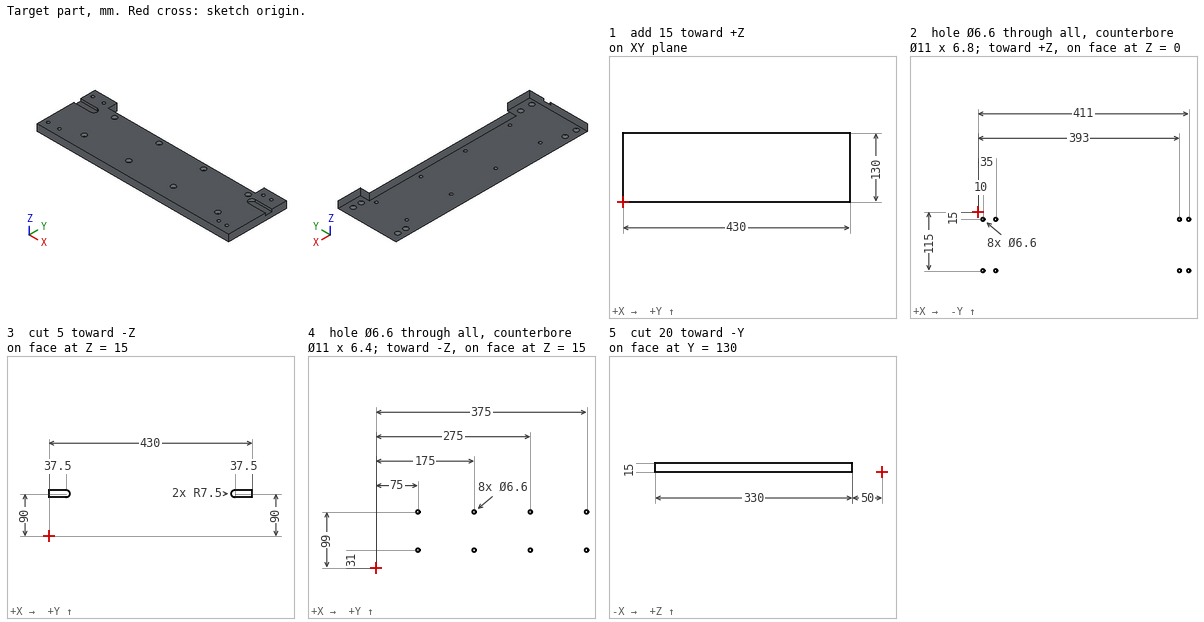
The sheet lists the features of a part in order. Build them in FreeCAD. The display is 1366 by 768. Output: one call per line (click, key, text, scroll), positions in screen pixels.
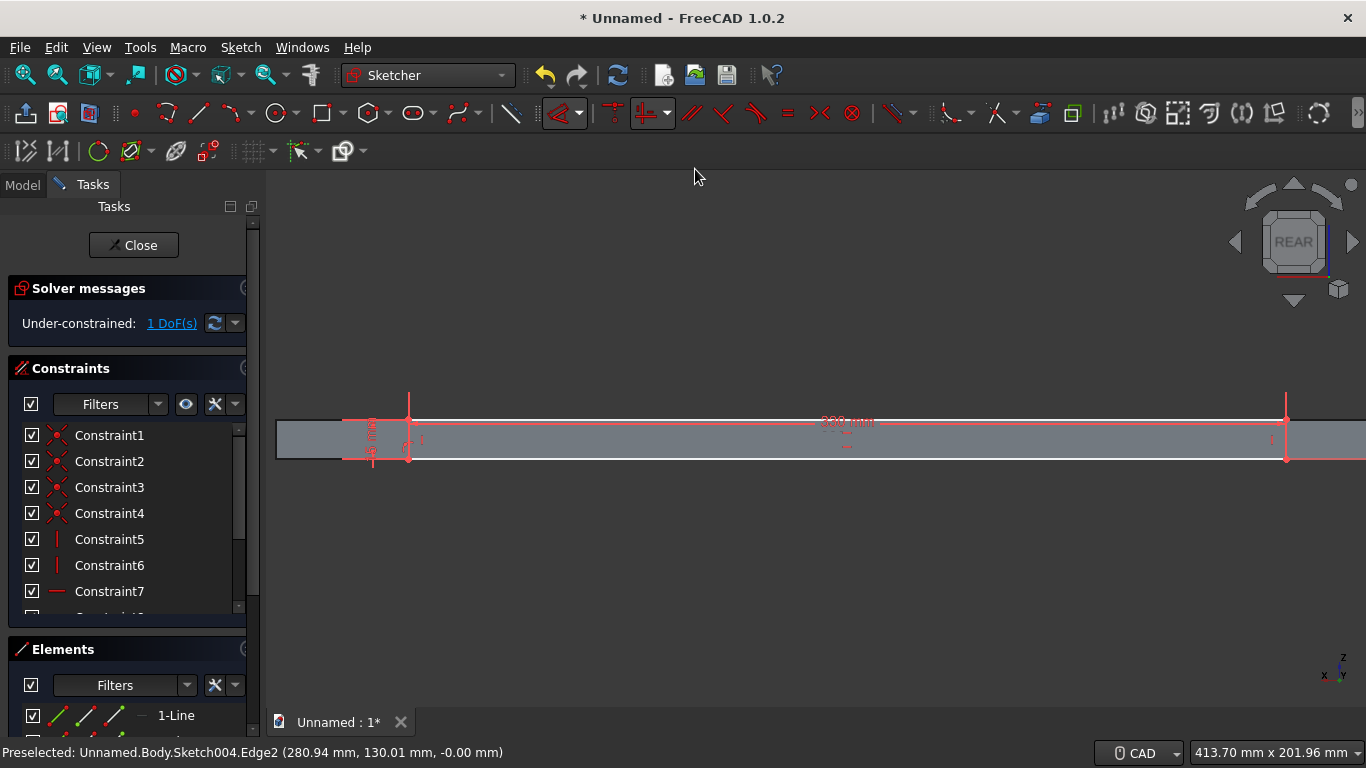
scroll(409, 436, down, 2)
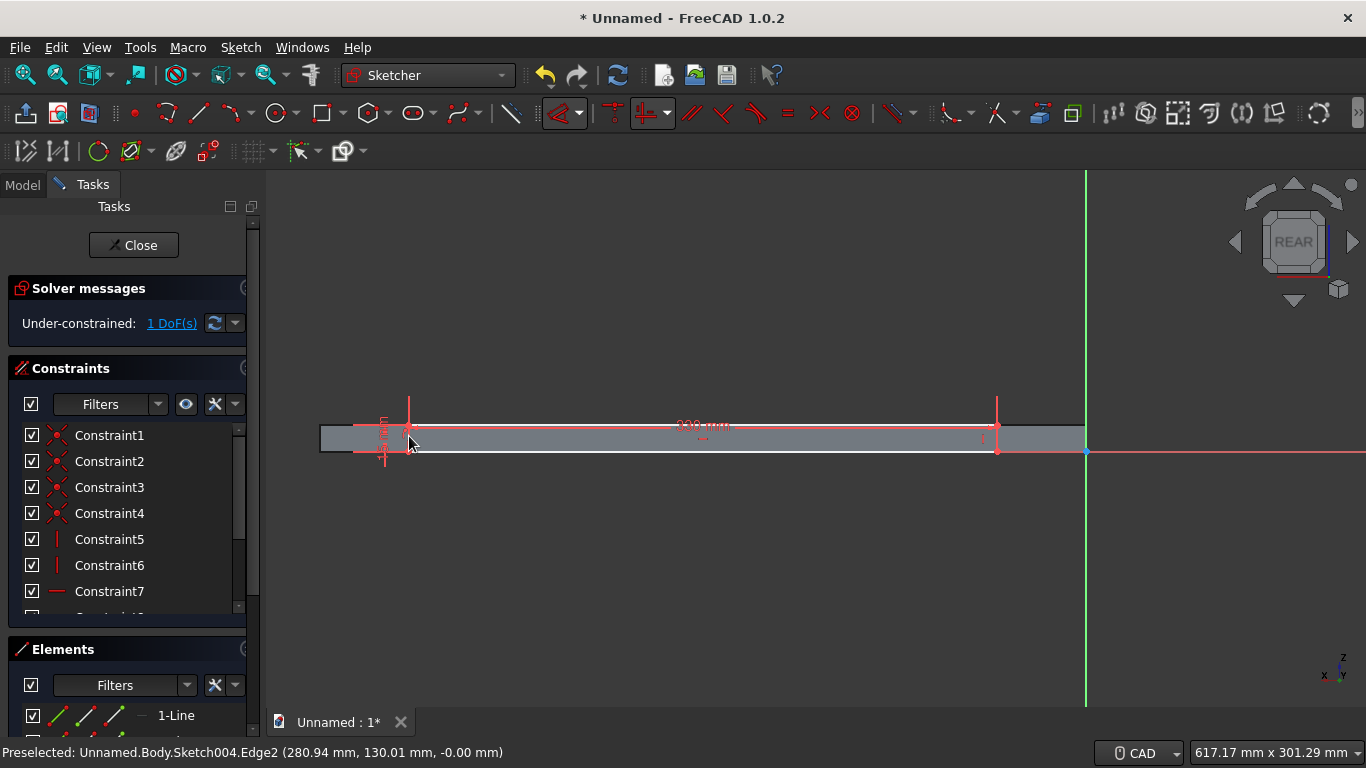
click(997, 452)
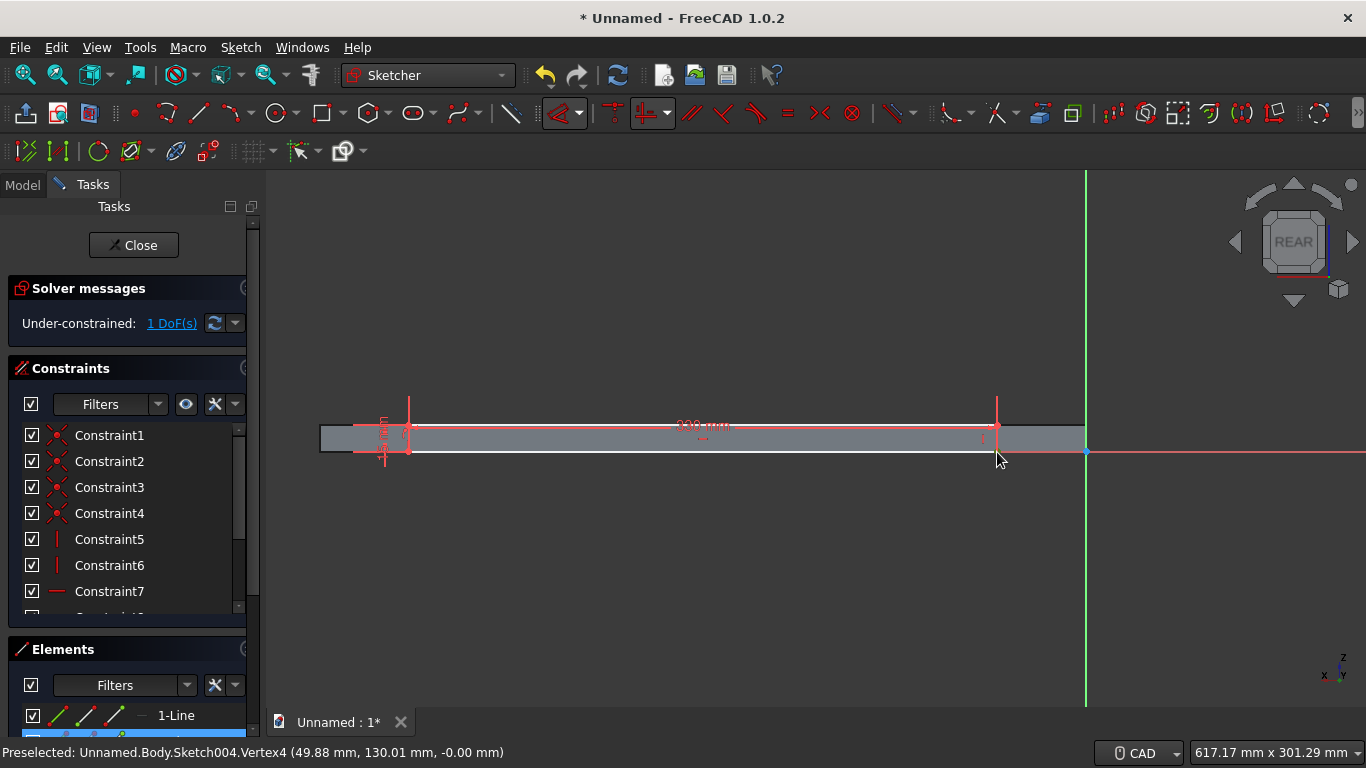
key(l)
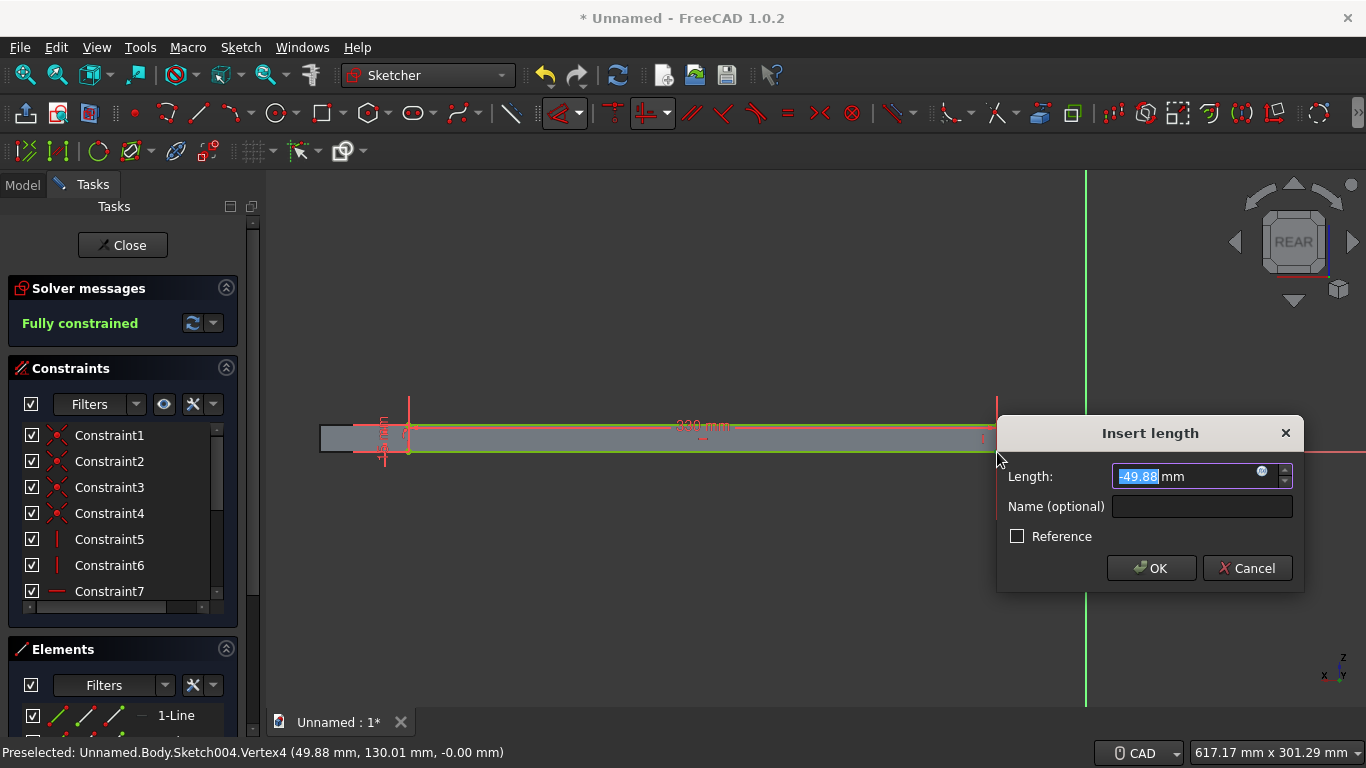
text(-50)
key(Return)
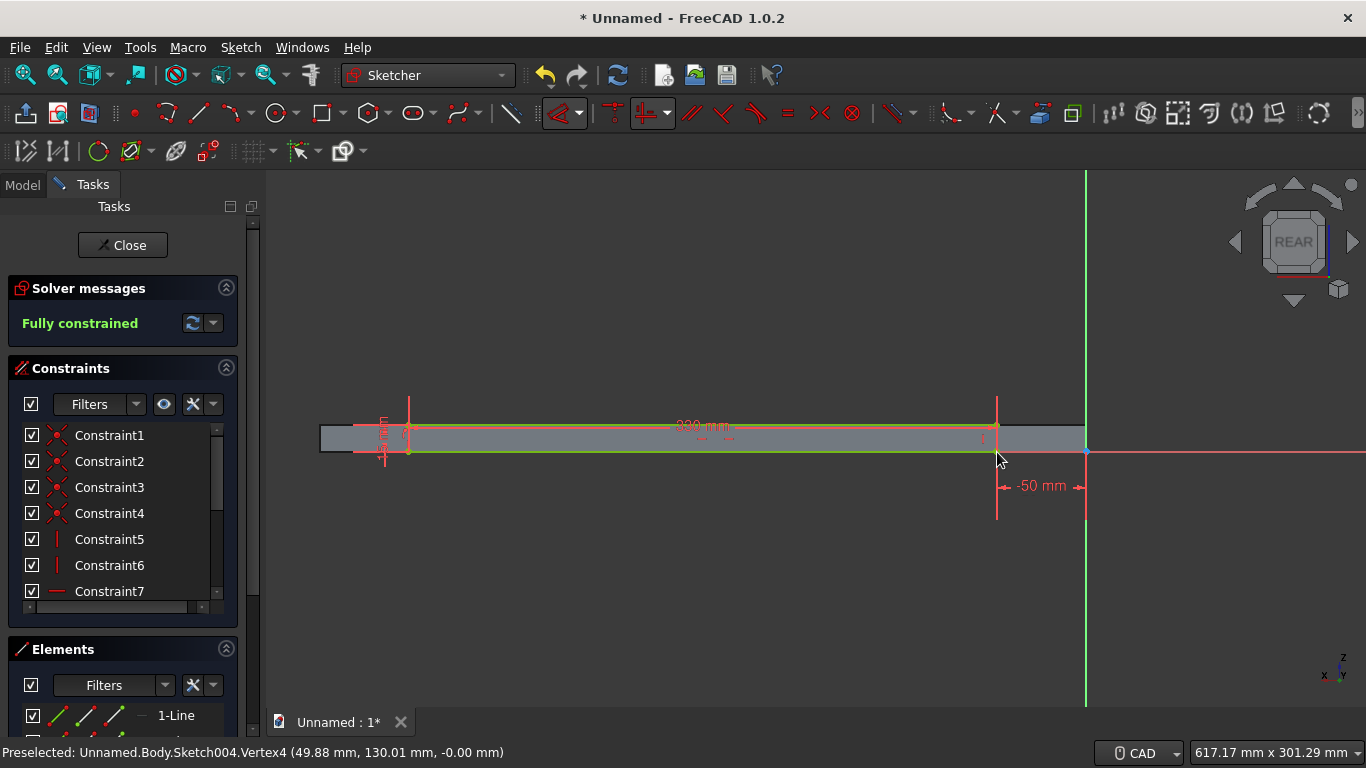
click(123, 245)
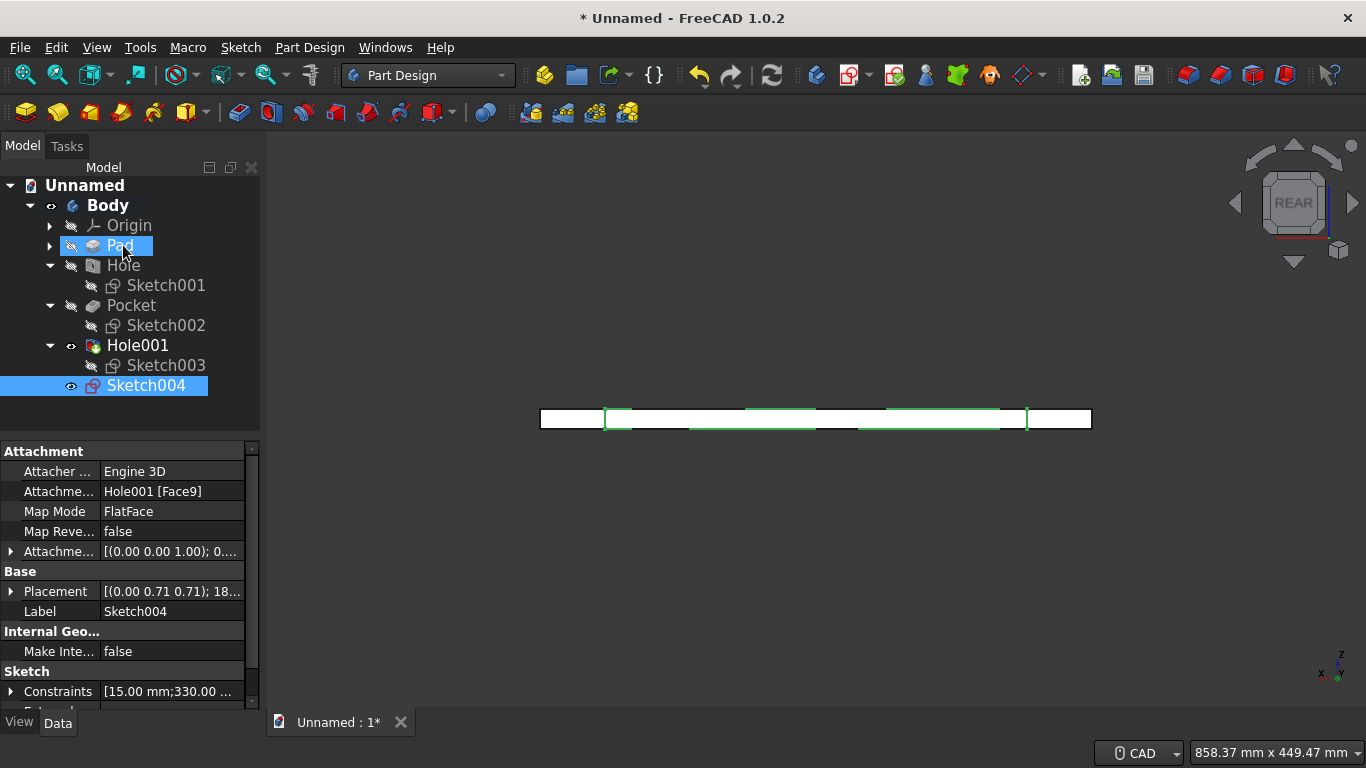
click(240, 112)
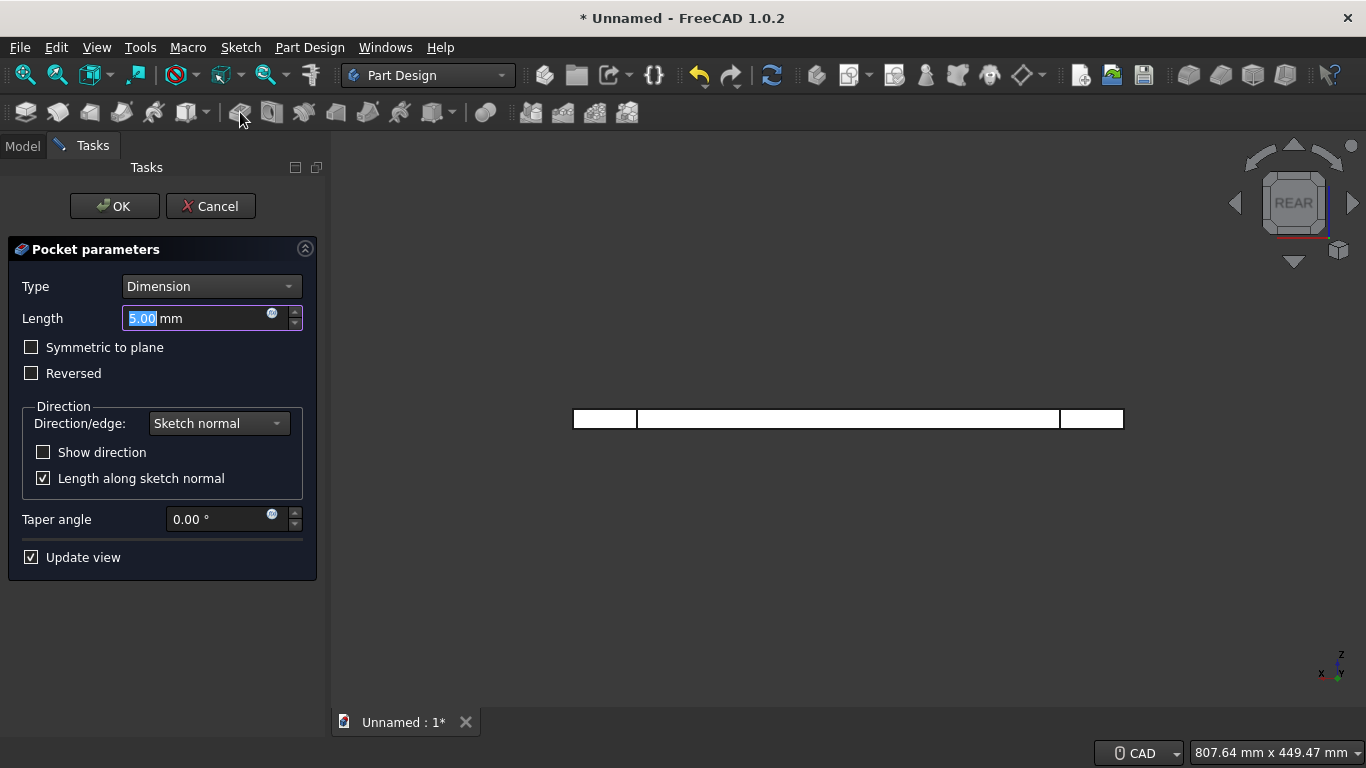
text(20)
key(Tab)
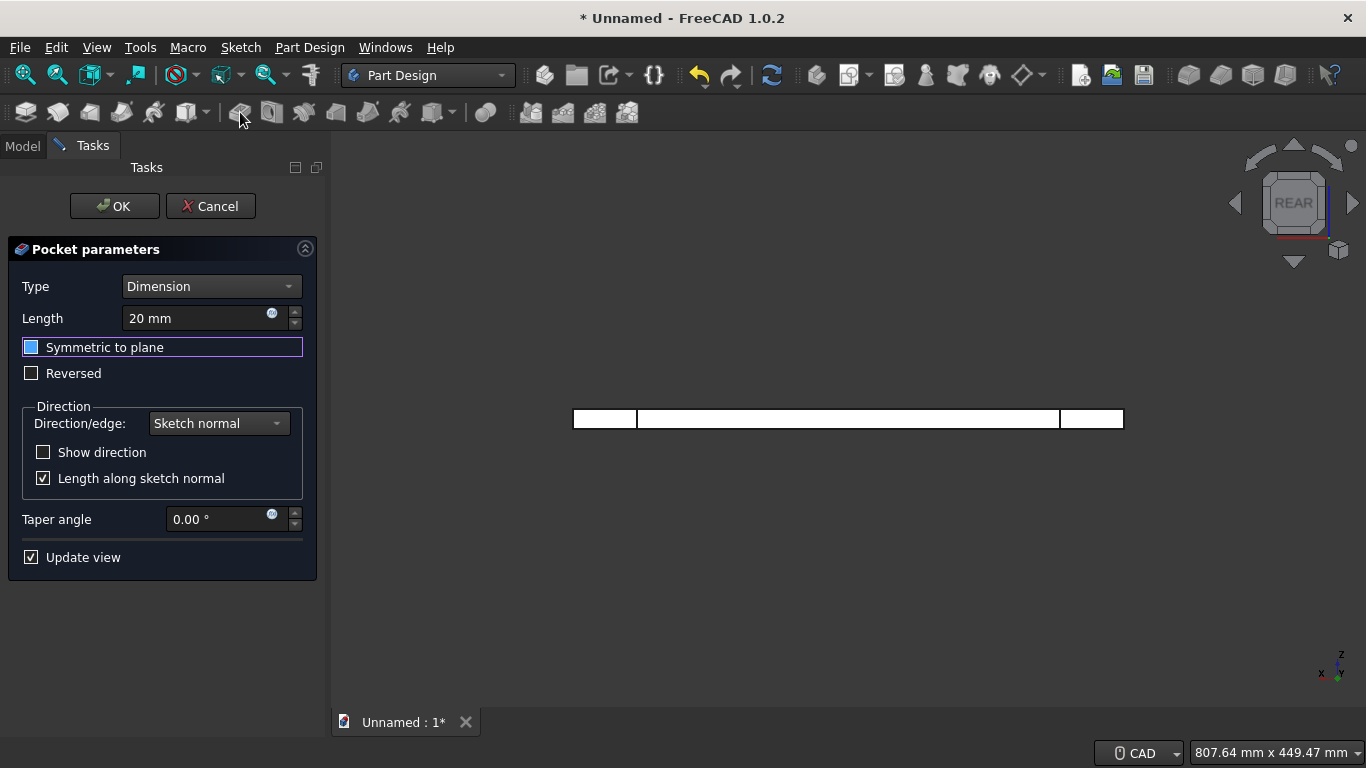
click(115, 206)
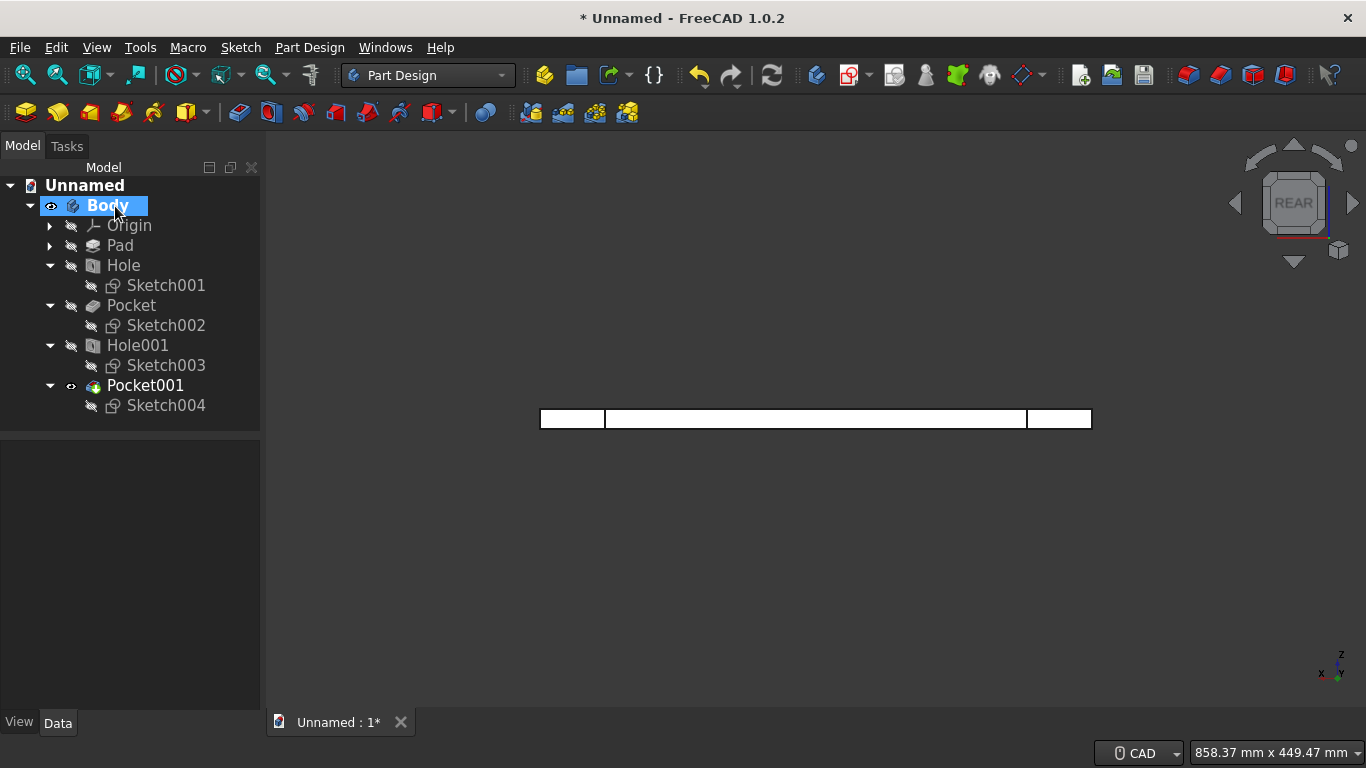
key(0)